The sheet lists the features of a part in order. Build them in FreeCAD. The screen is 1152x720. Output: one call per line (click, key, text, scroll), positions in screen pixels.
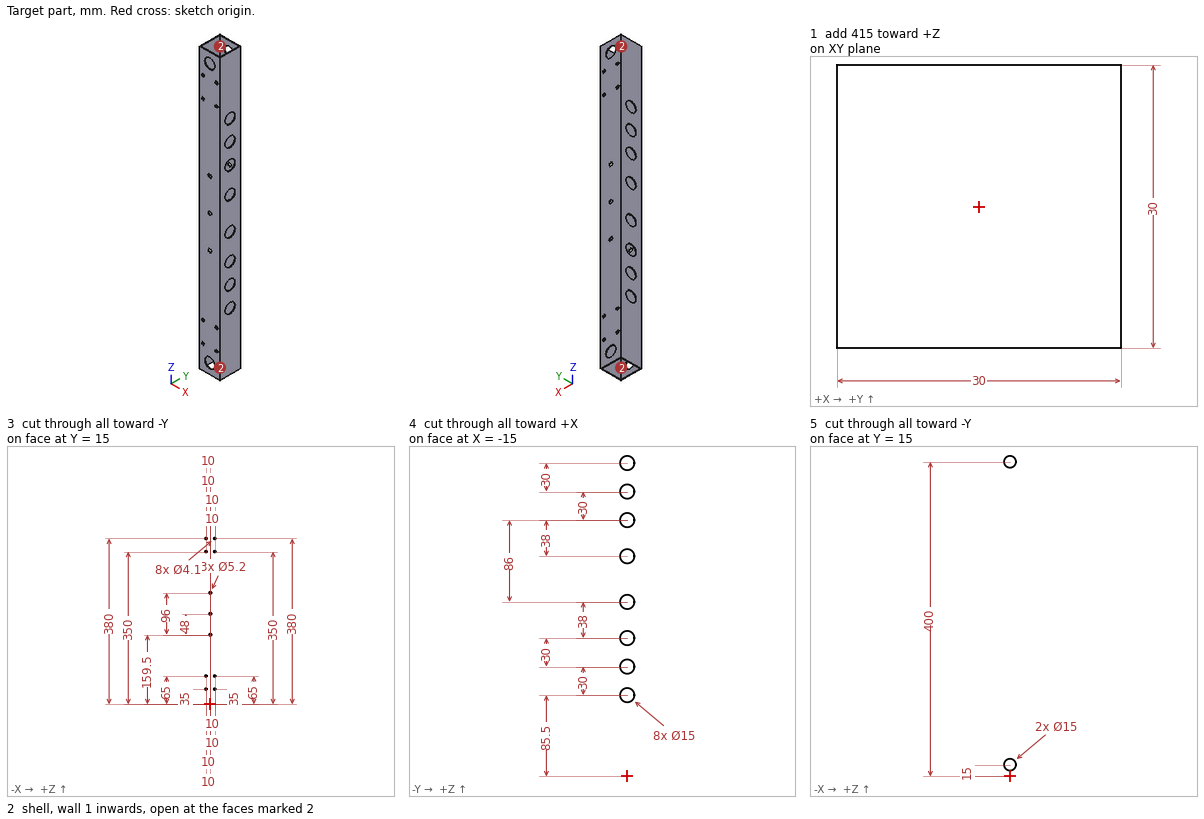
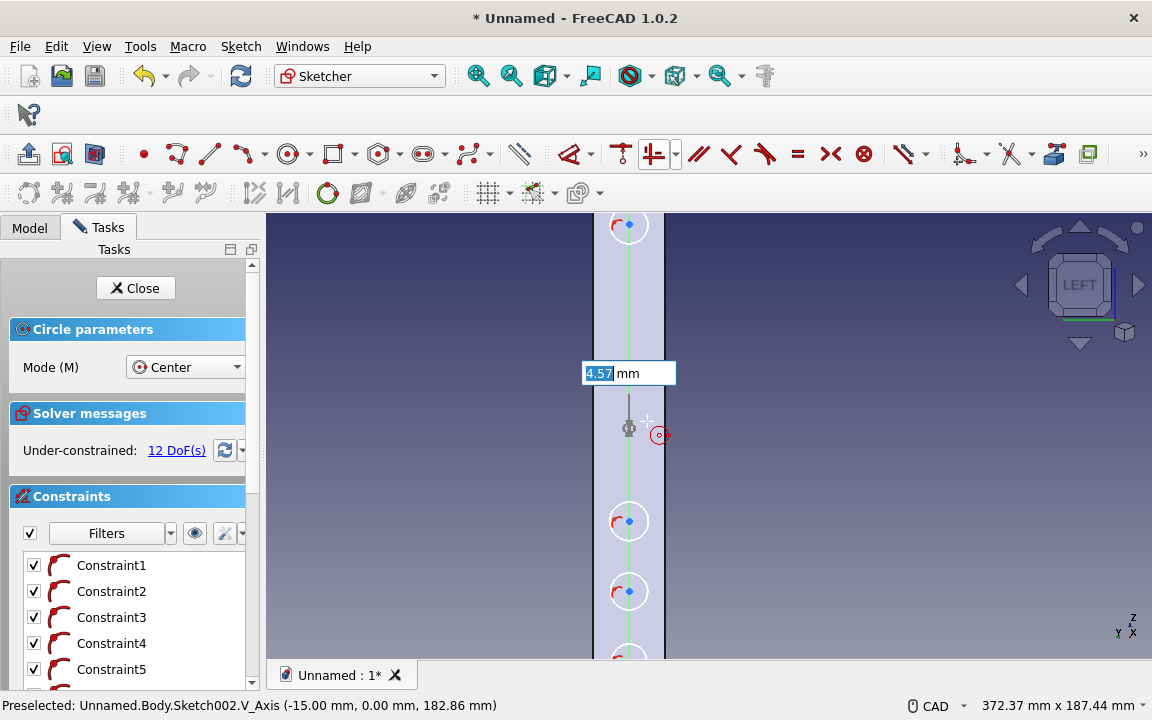
click(646, 421)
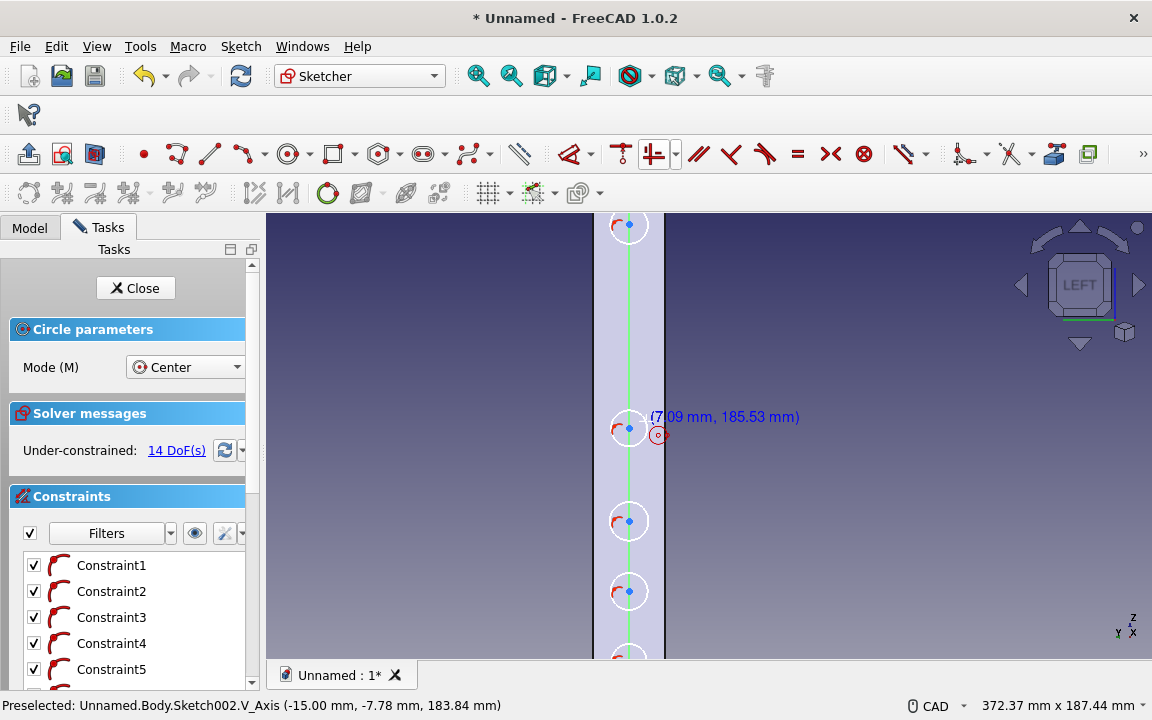
scroll(629, 313, up, 2)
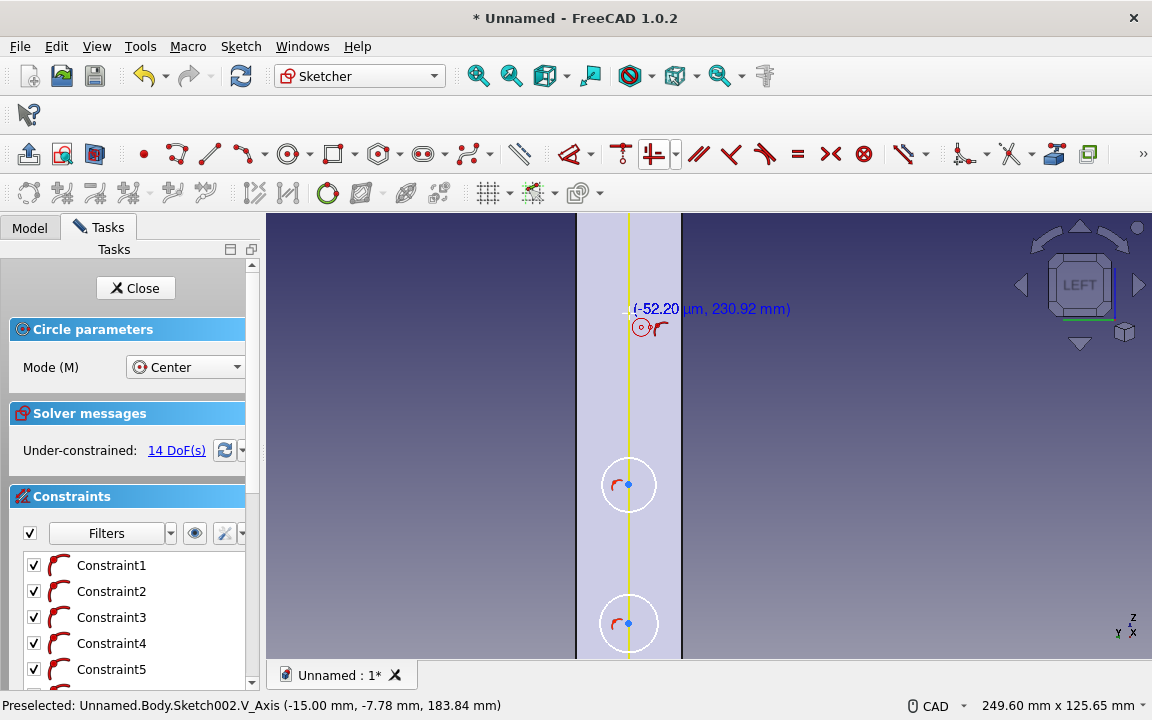
scroll(644, 403, down, 7)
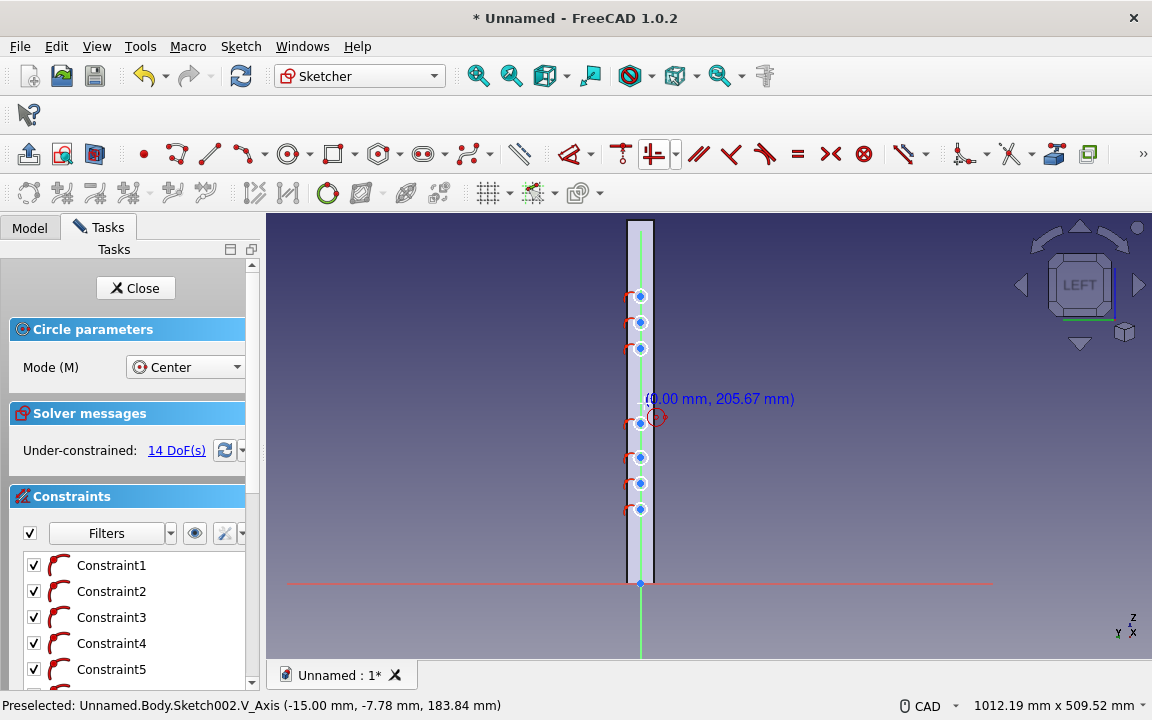
click(641, 381)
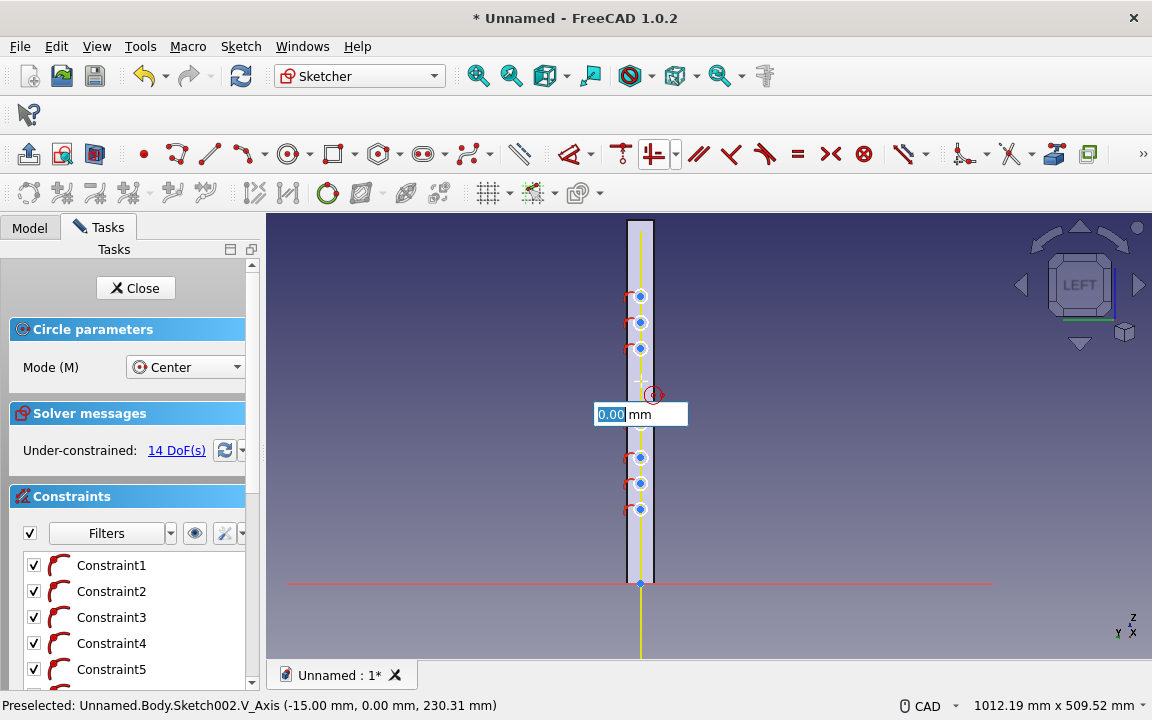
scroll(647, 379, up, 5)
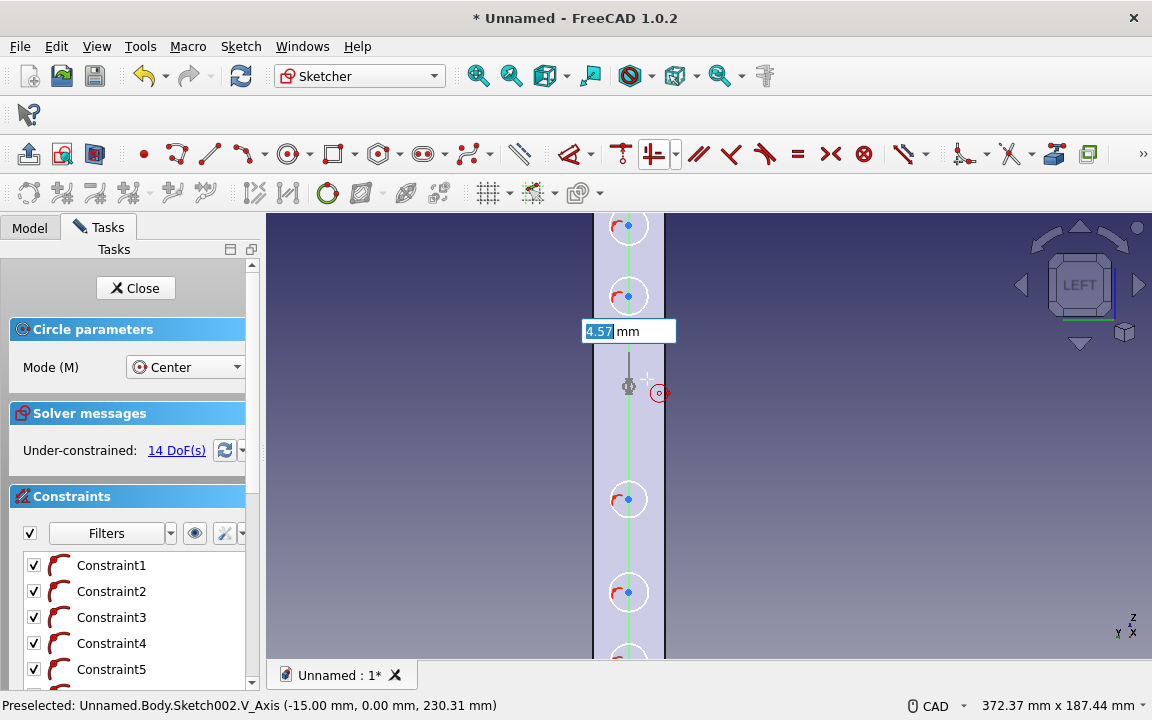
click(646, 378)
key(Escape)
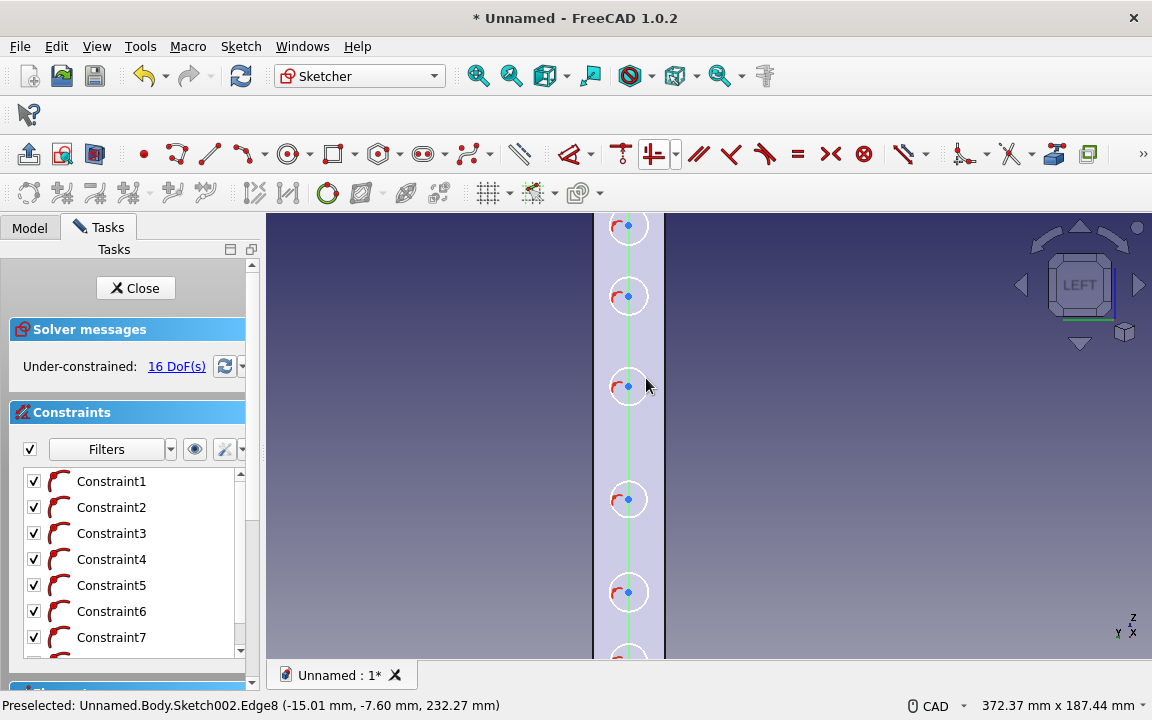
scroll(647, 379, down, 5)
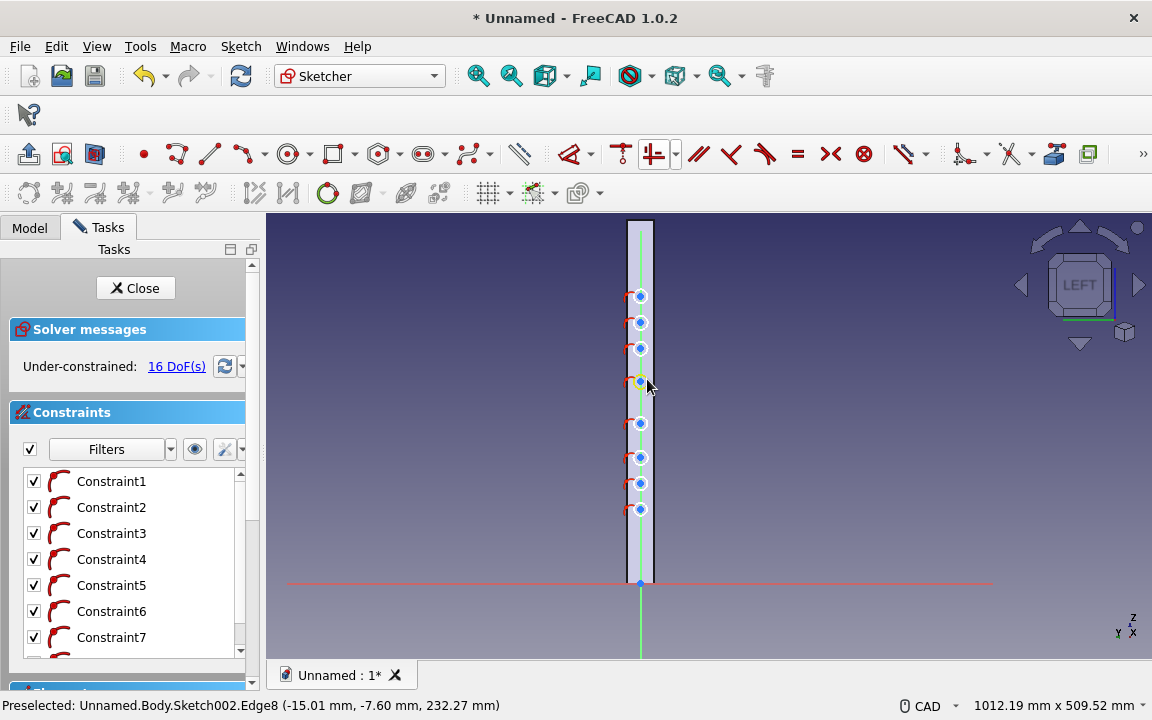
scroll(645, 505, up, 6)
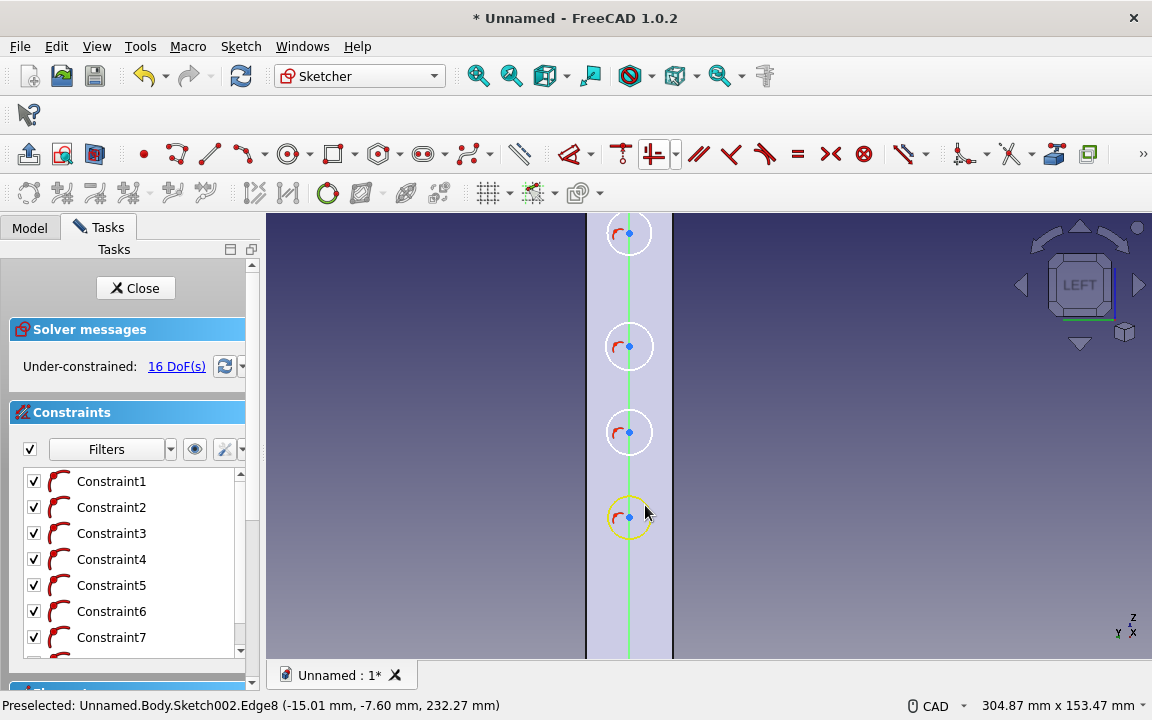
click(645, 503)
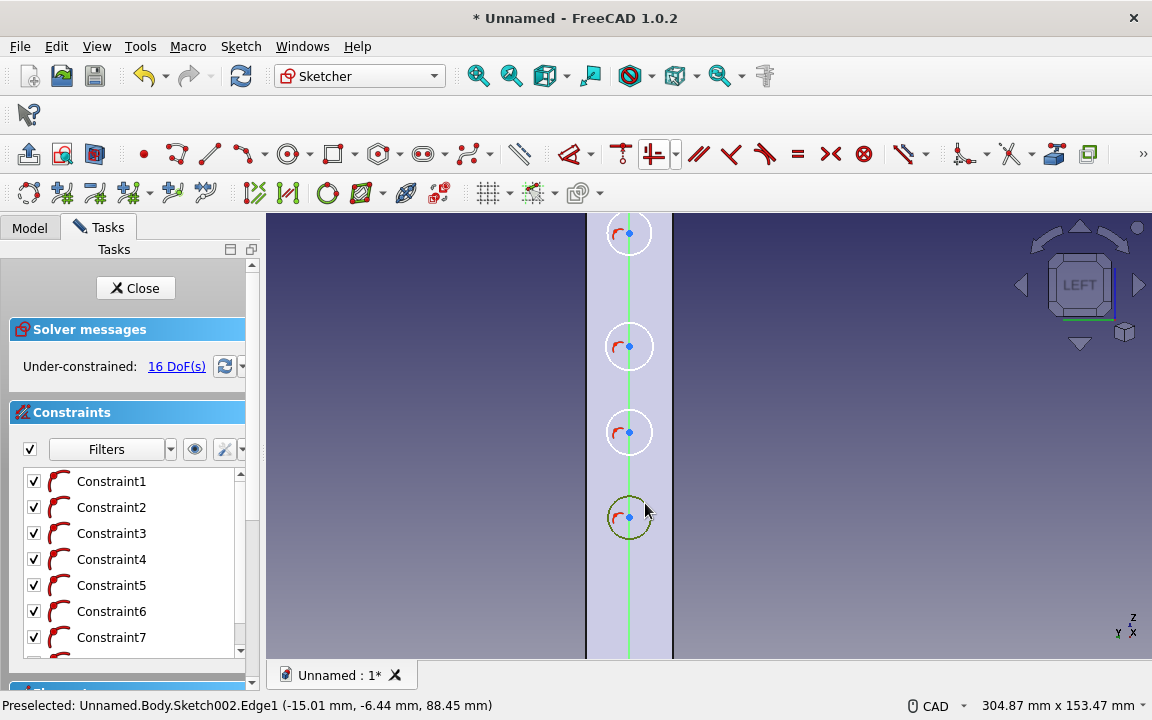
click(645, 416)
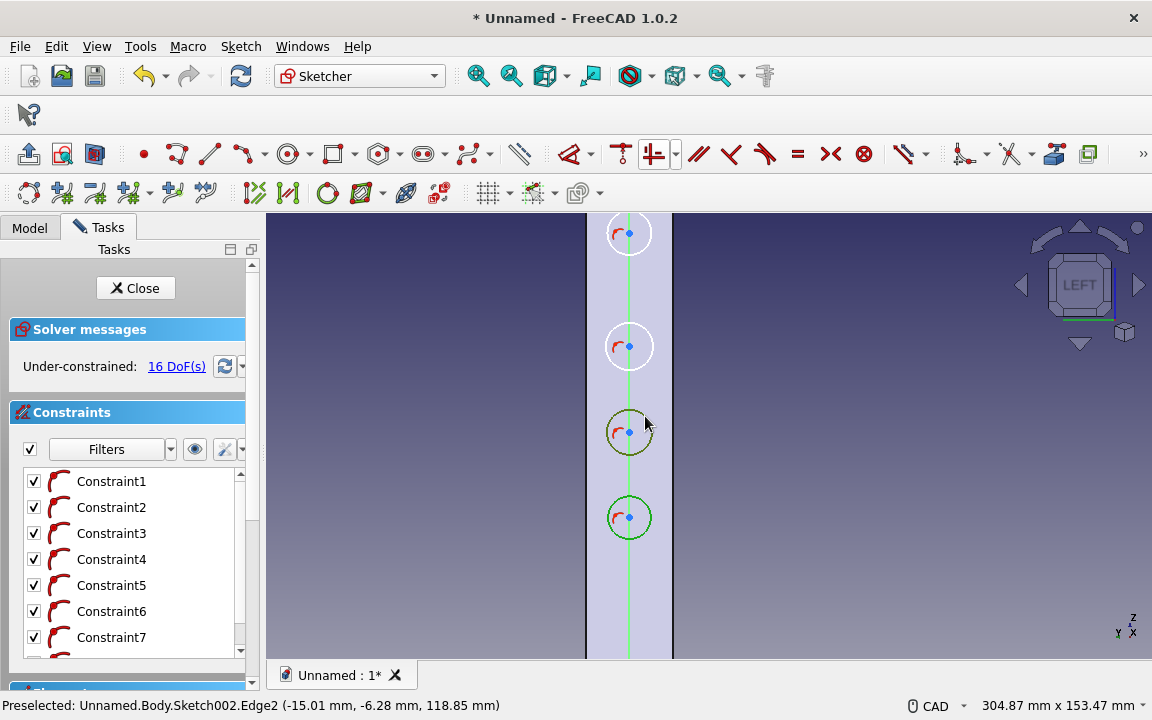
click(646, 330)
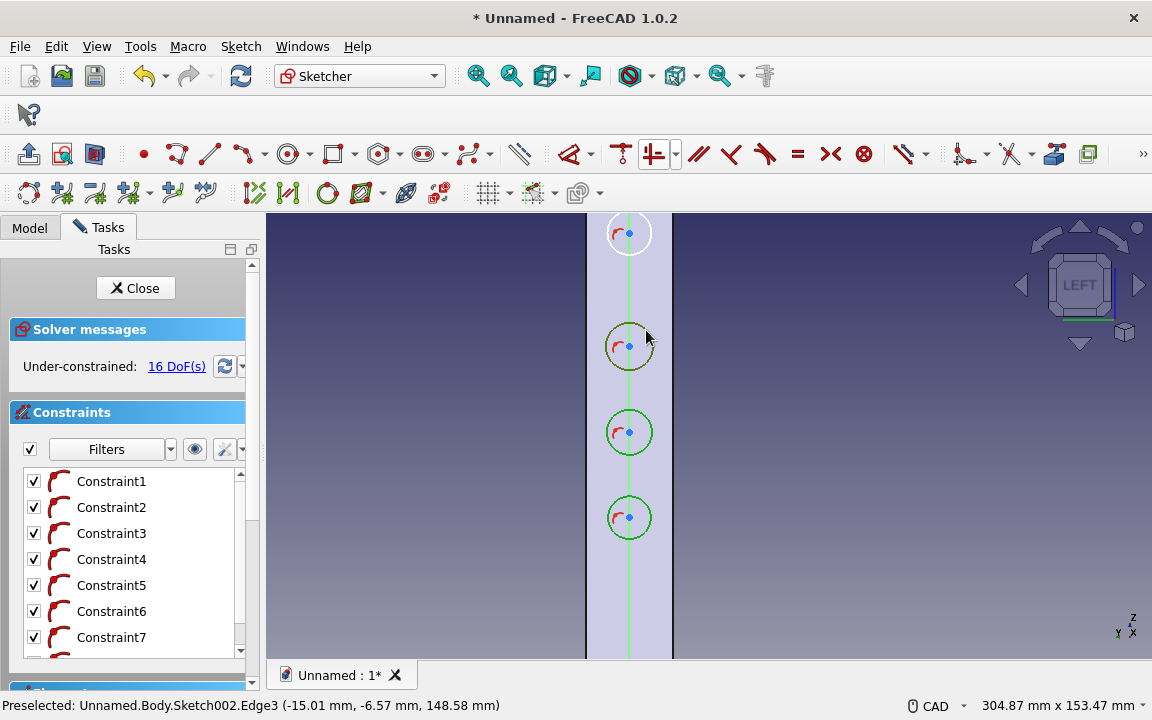
scroll(645, 506, down, 6)